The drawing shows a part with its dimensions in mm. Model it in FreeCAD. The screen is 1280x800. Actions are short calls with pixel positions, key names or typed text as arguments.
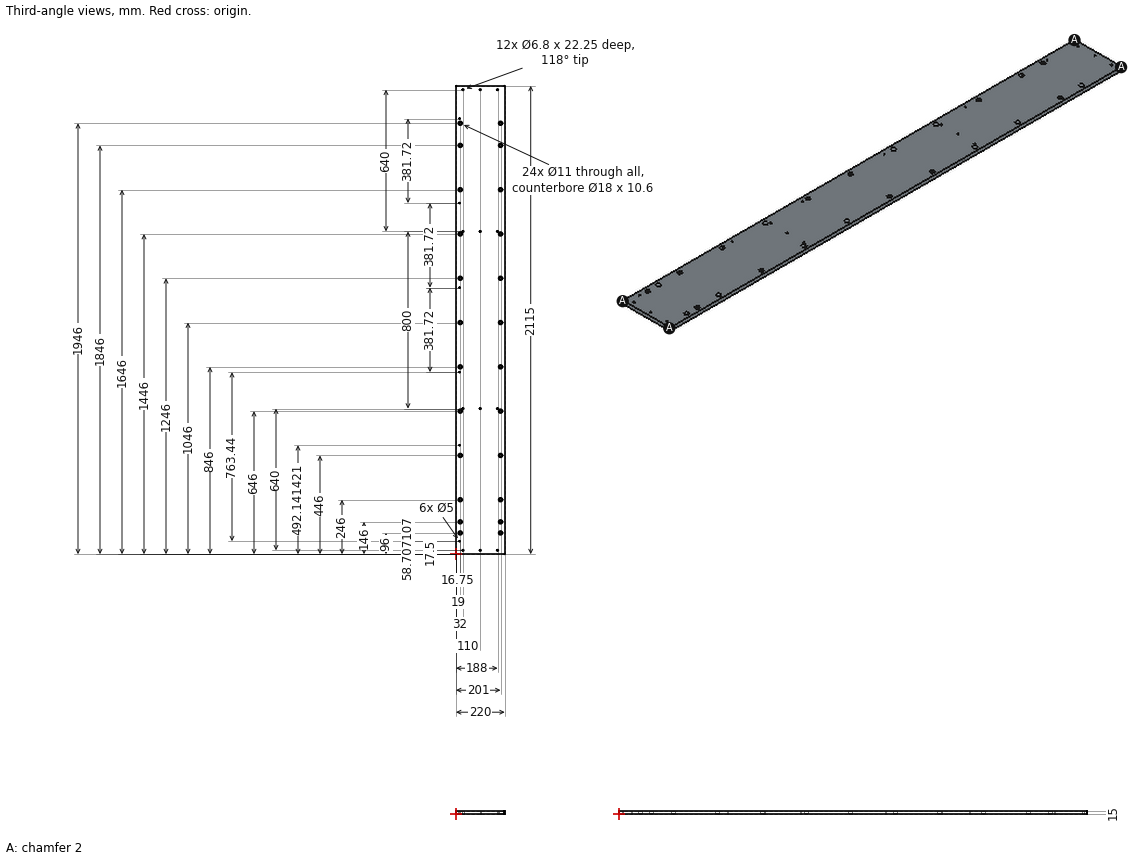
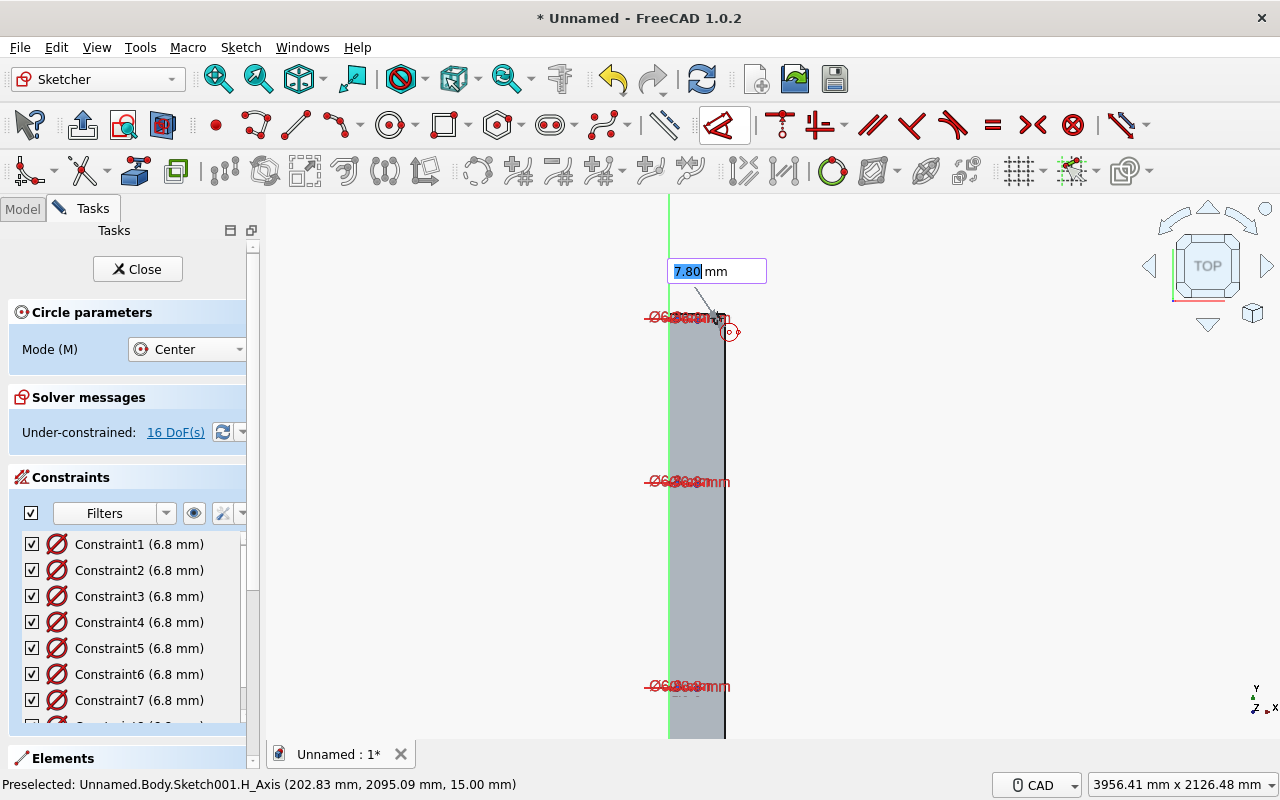
text(6.8)
key(Return)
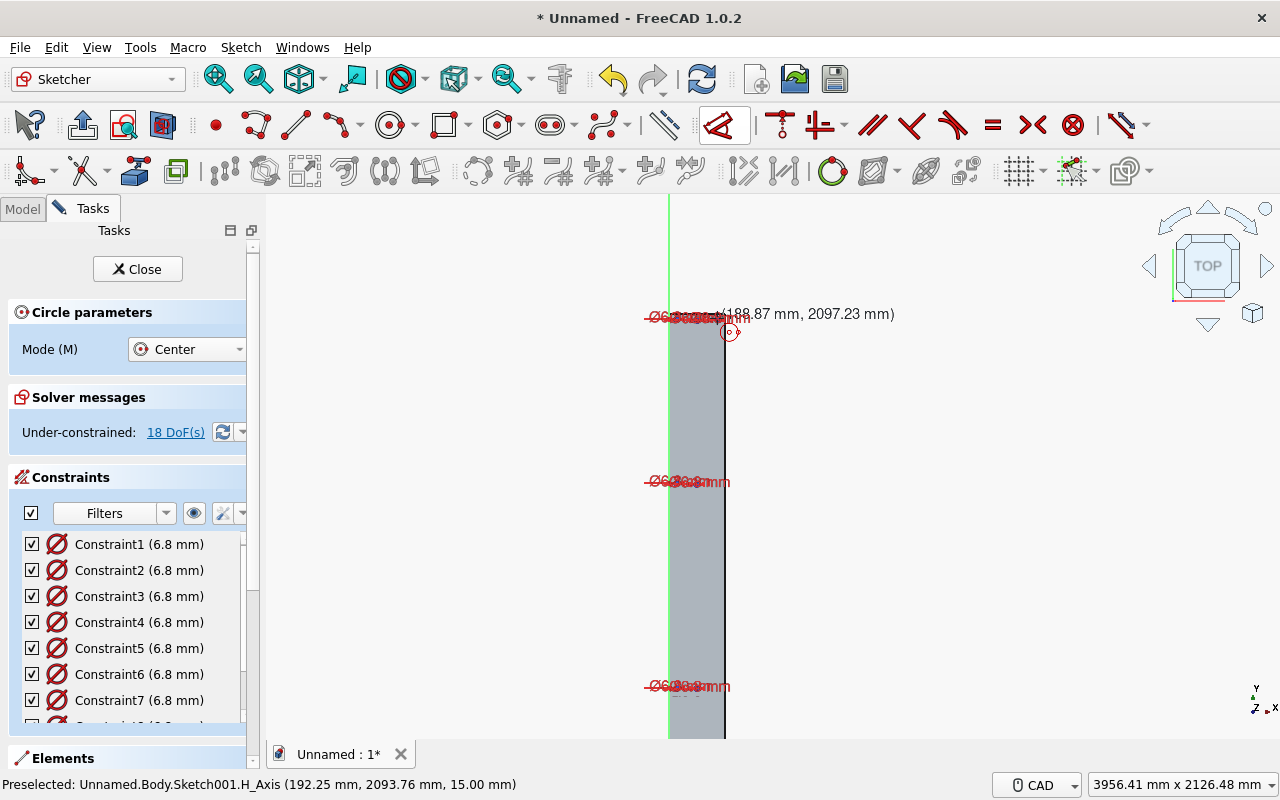
scroll(717, 483, up, 17)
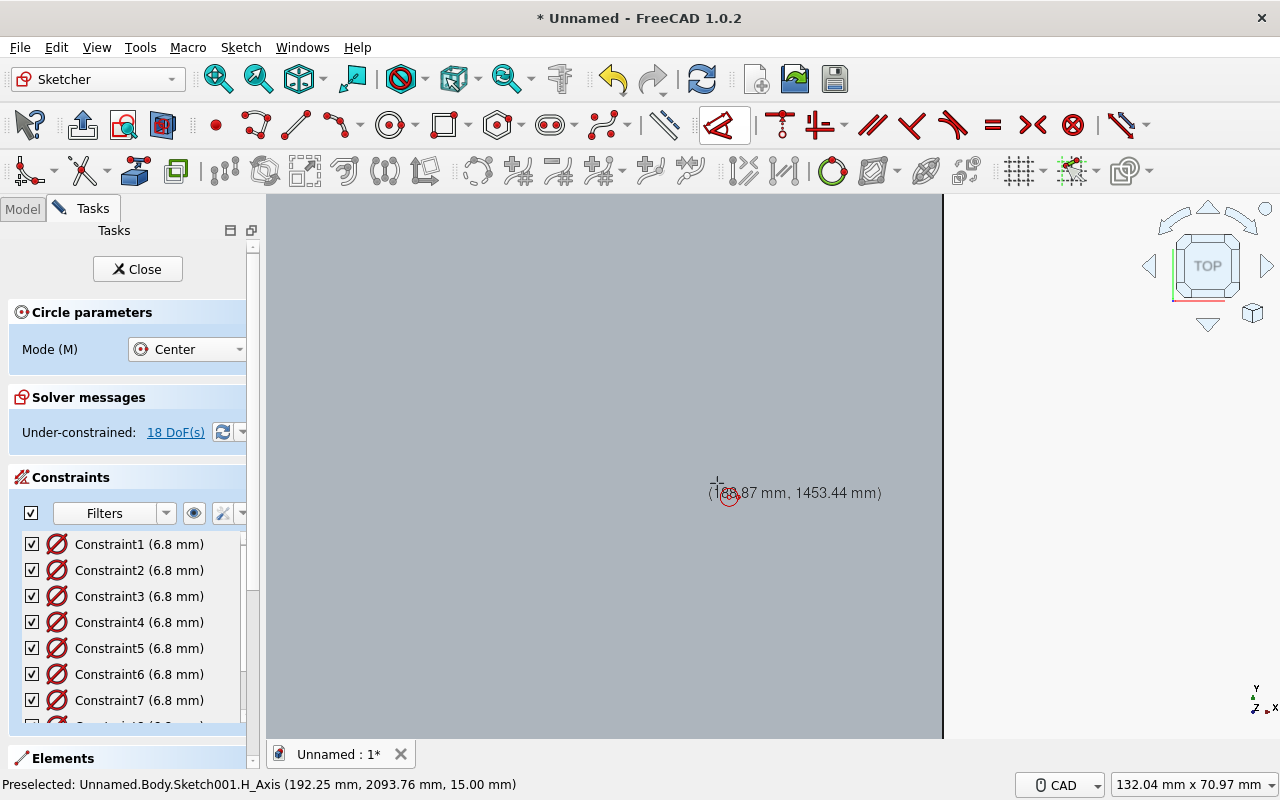
scroll(704, 466, down, 15)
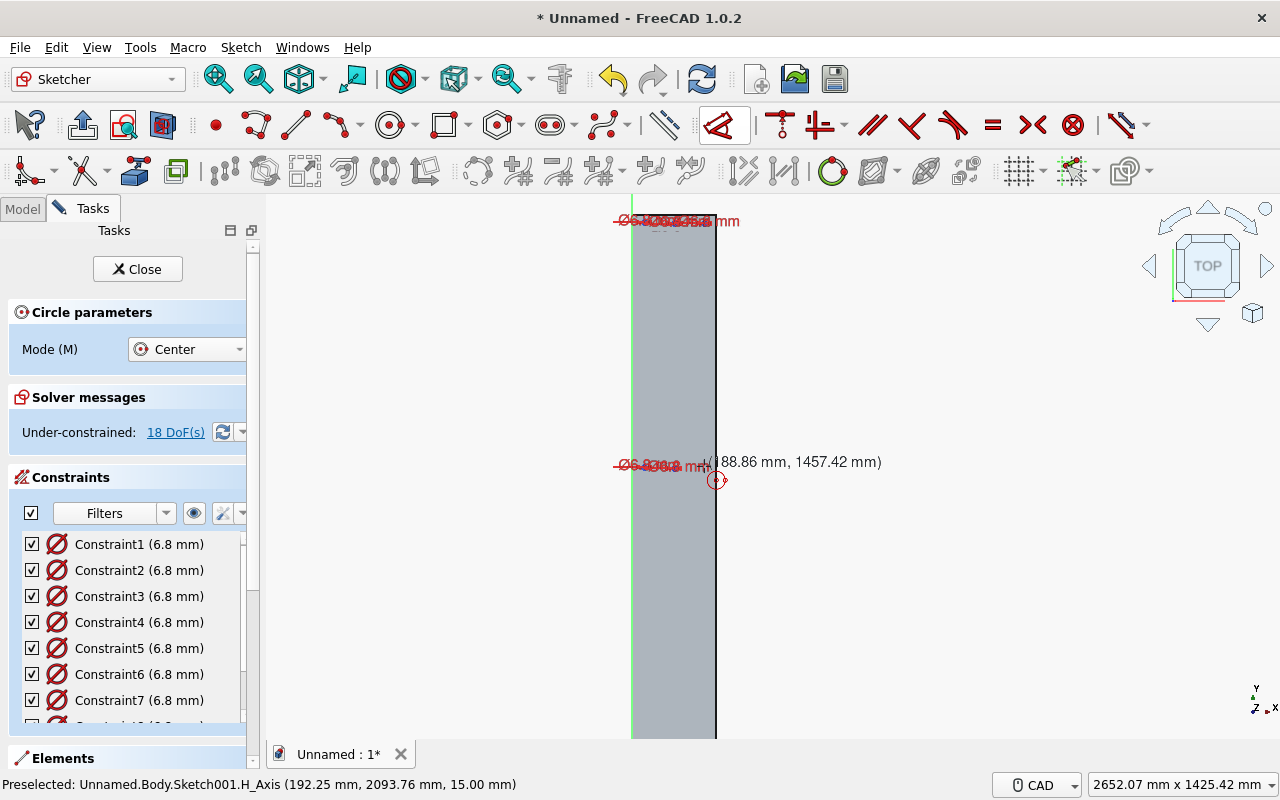
scroll(734, 340, down, 4)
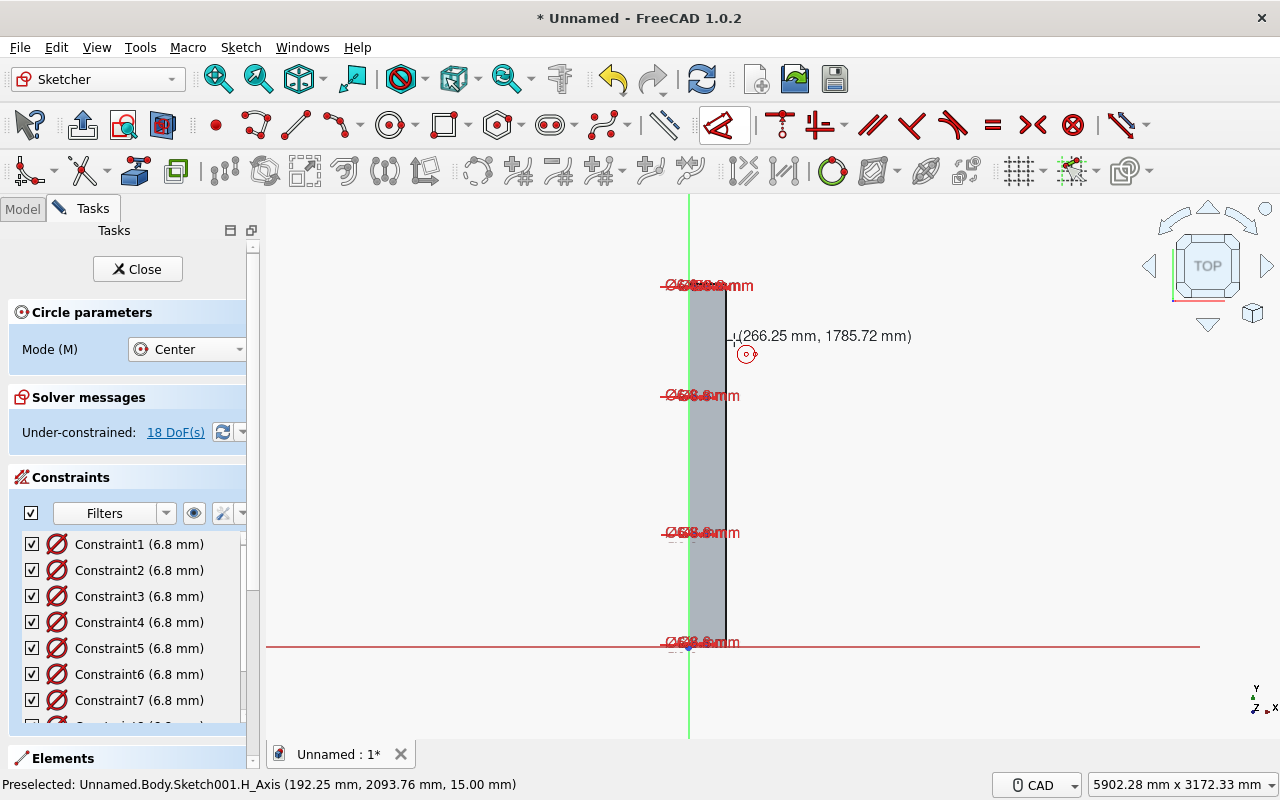
scroll(721, 397, up, 2)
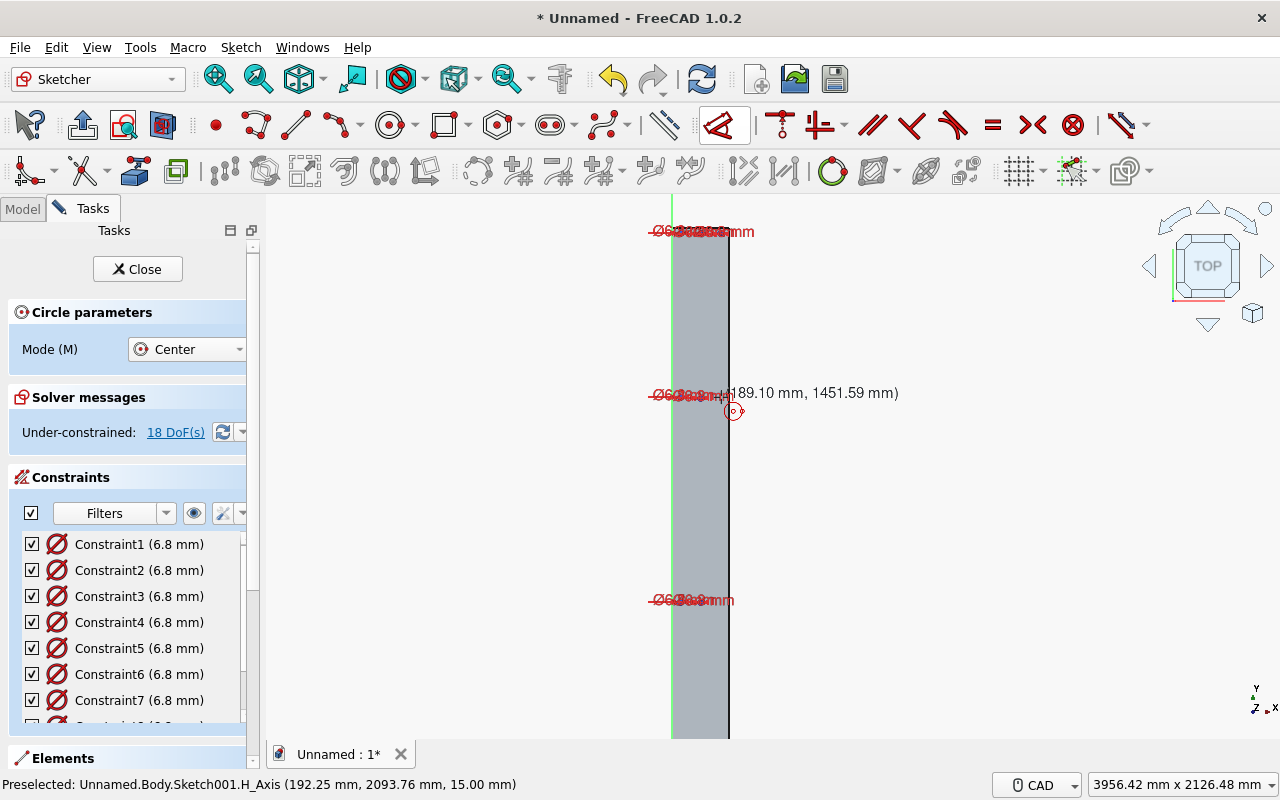
click(720, 397)
move(721, 396)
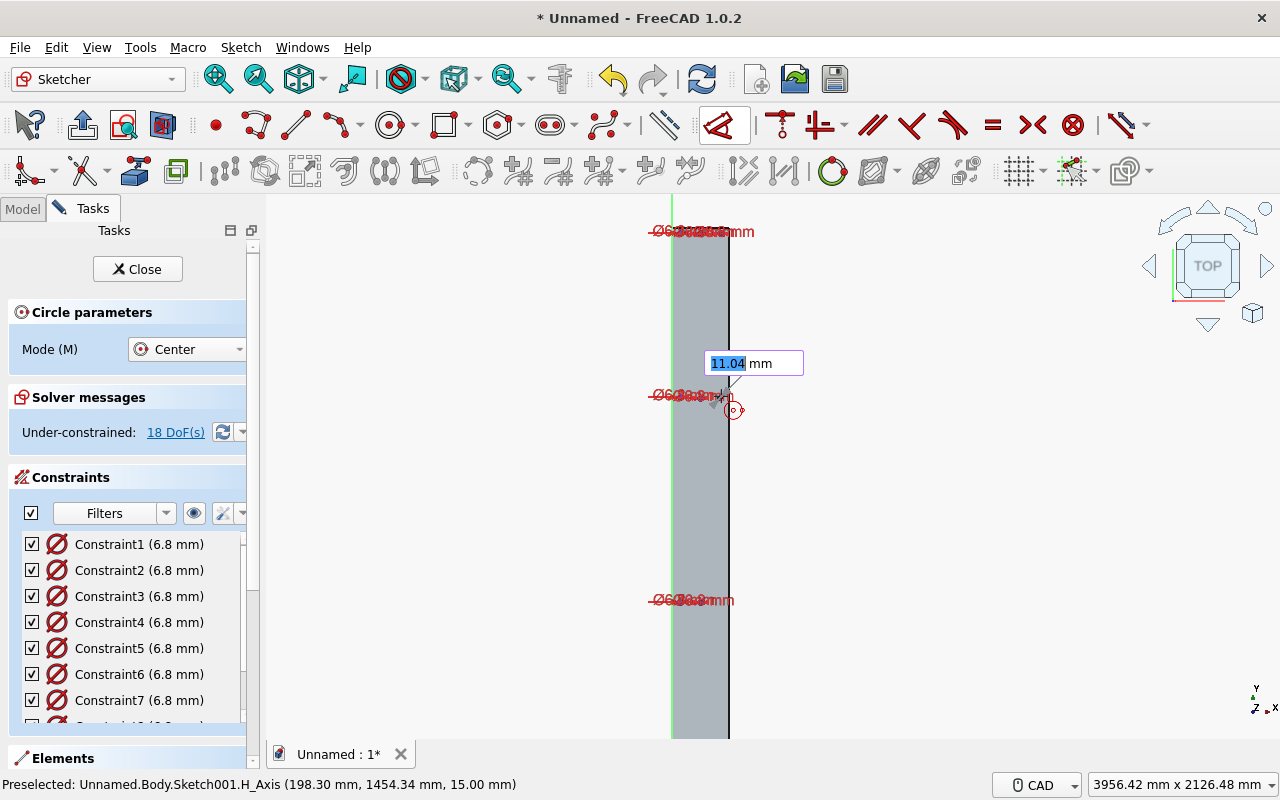
text(6.8)
key(Return)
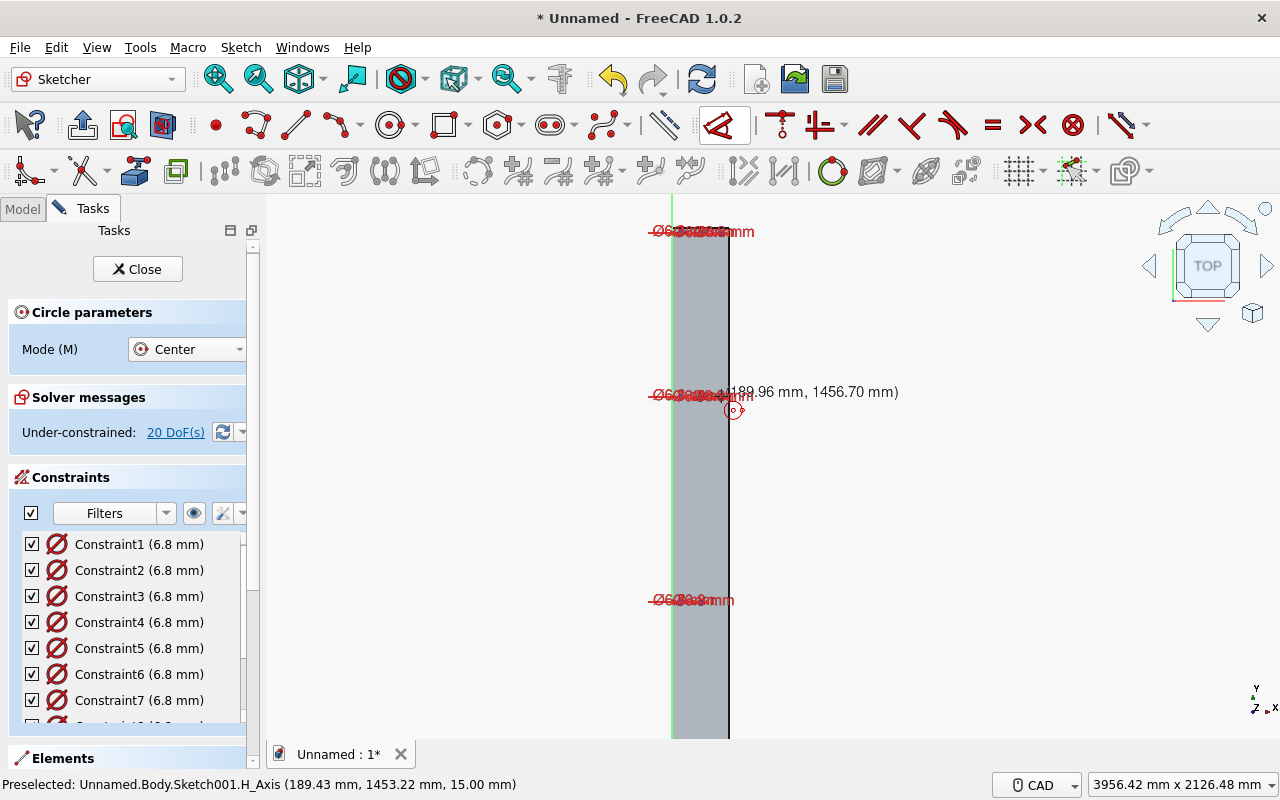
scroll(720, 602, up, 17)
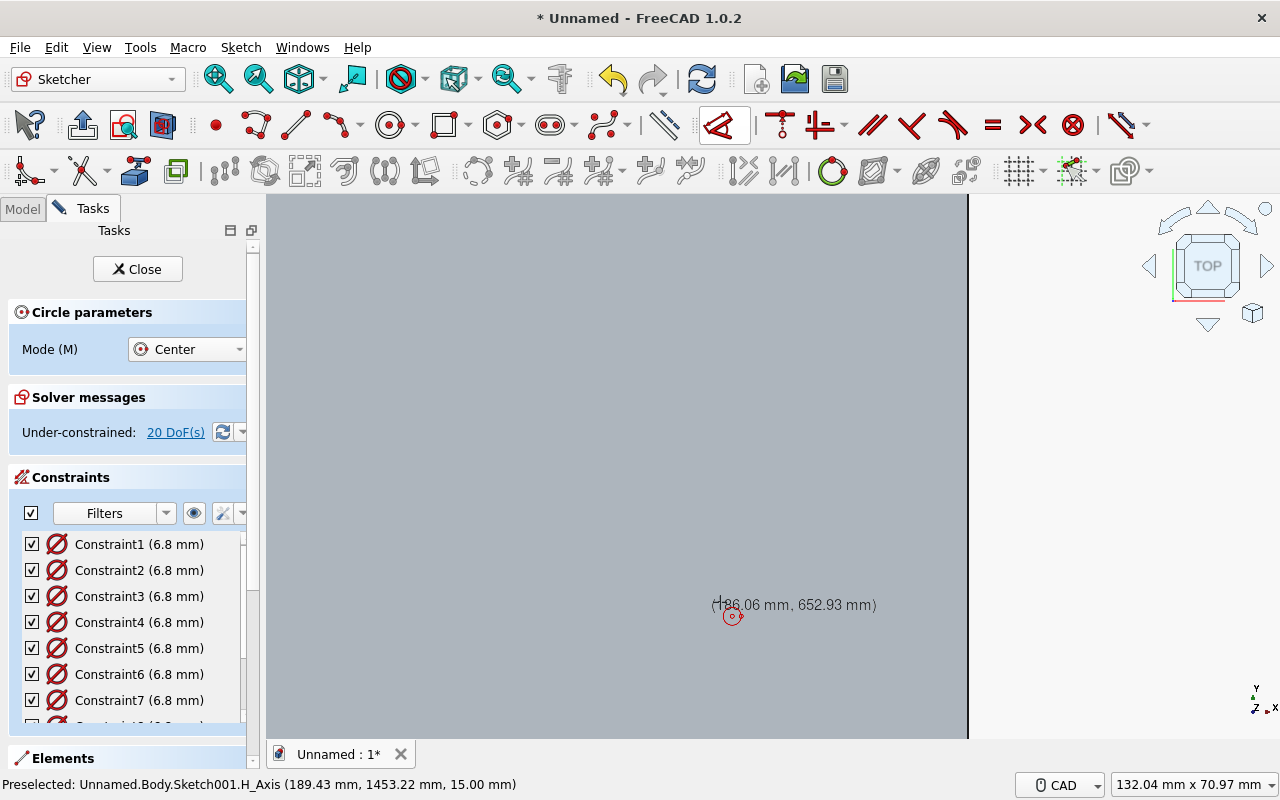
scroll(704, 466, down, 15)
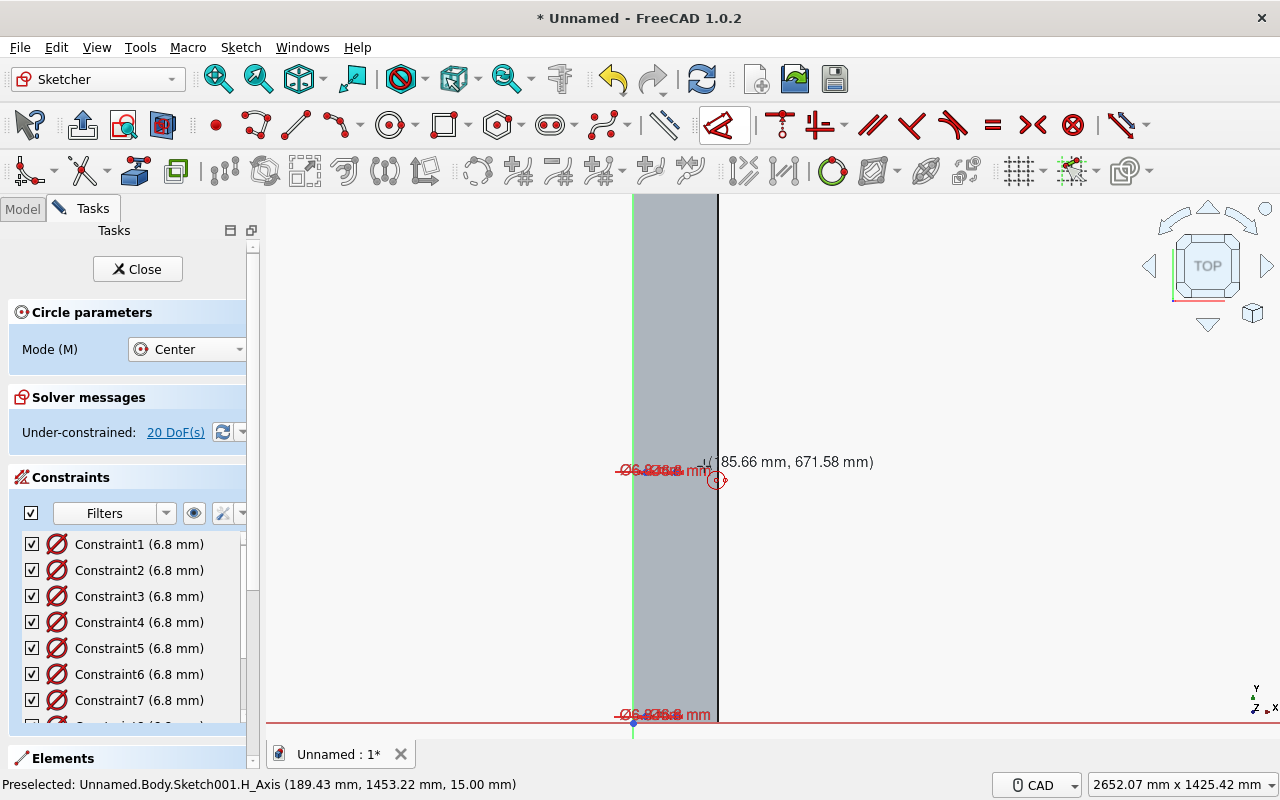
scroll(733, 585, down, 4)